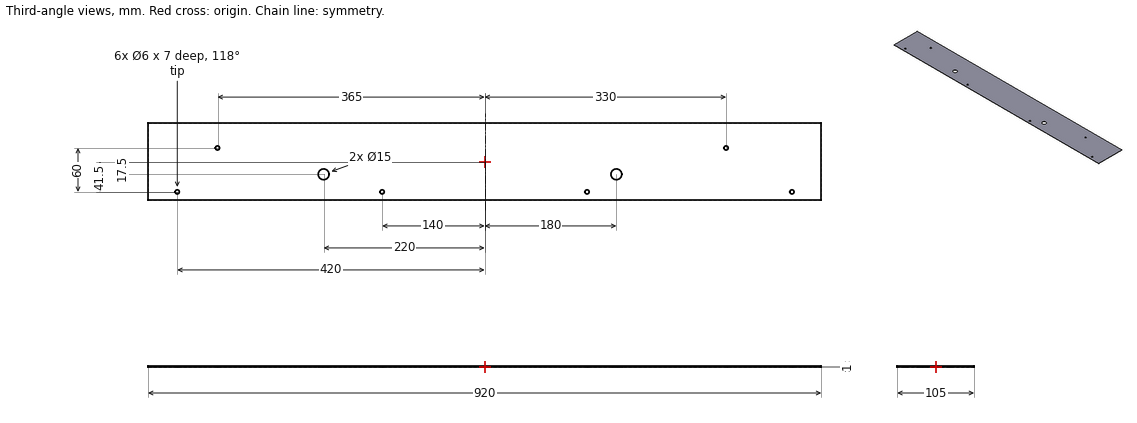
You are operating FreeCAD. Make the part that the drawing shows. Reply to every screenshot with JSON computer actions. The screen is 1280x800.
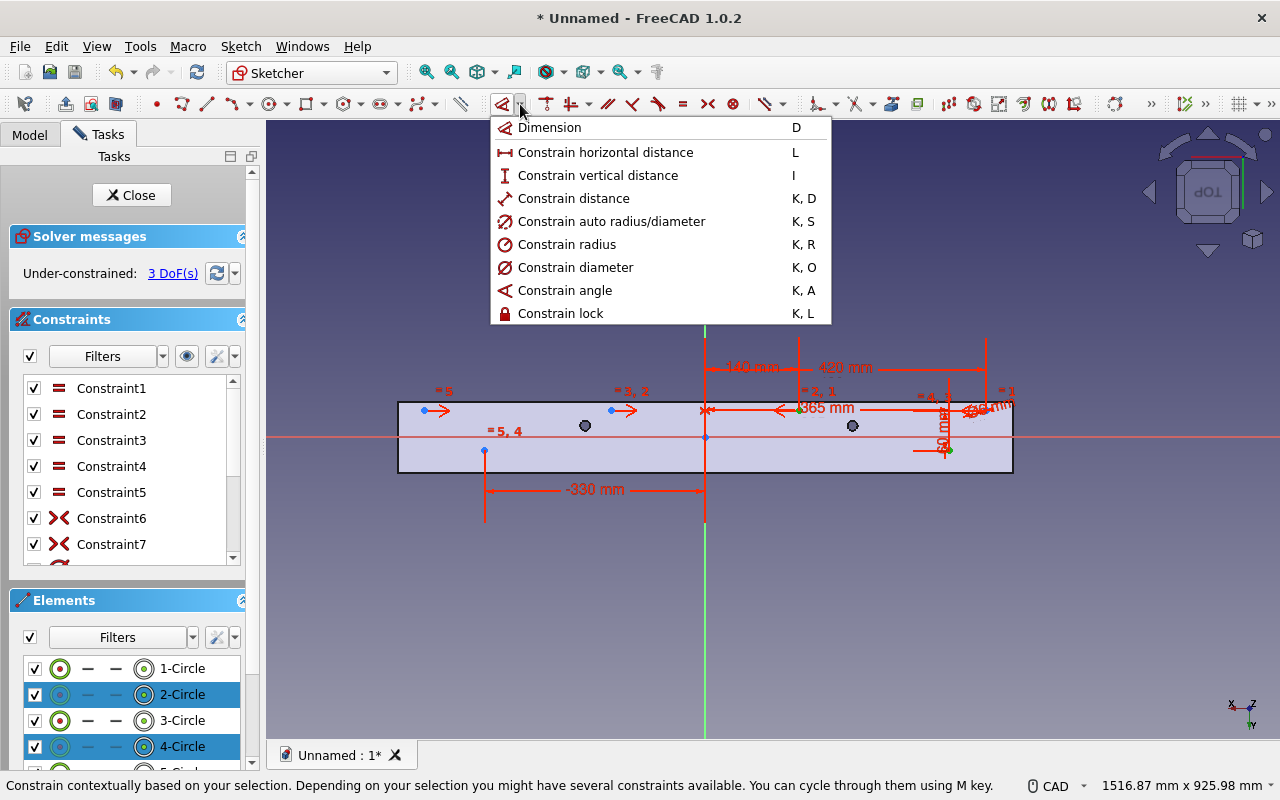
{"action": "left_click", "coordinate": [661, 176]}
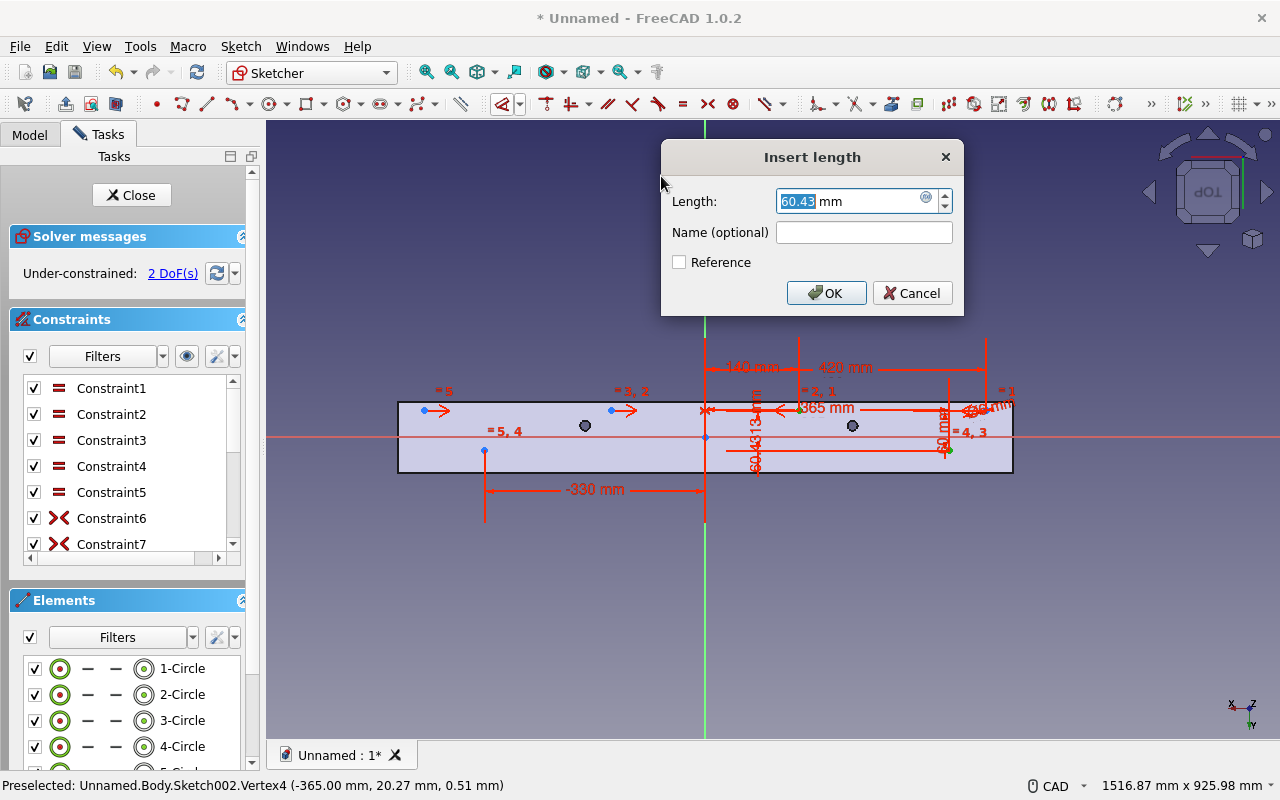
{"action": "type", "text": "60"}
{"action": "key", "text": "Return"}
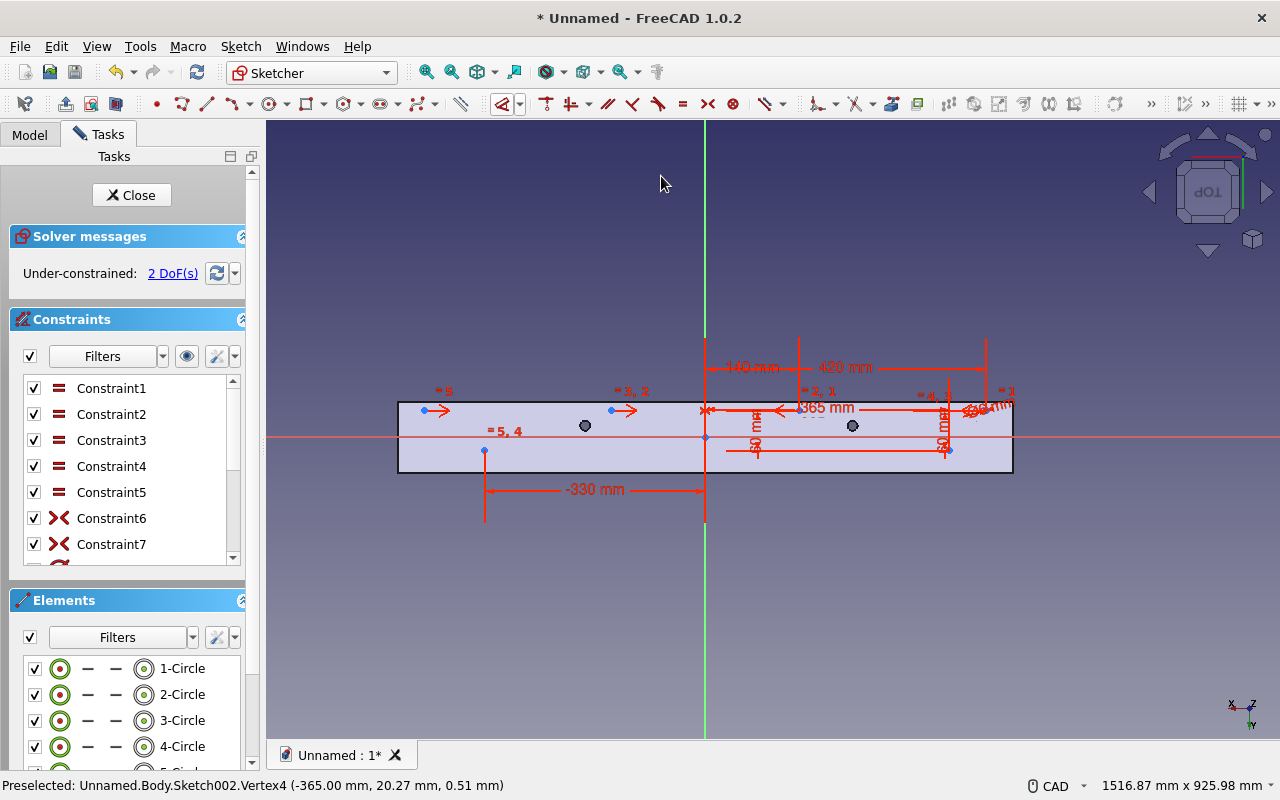
{"action": "left_click", "coordinate": [612, 411]}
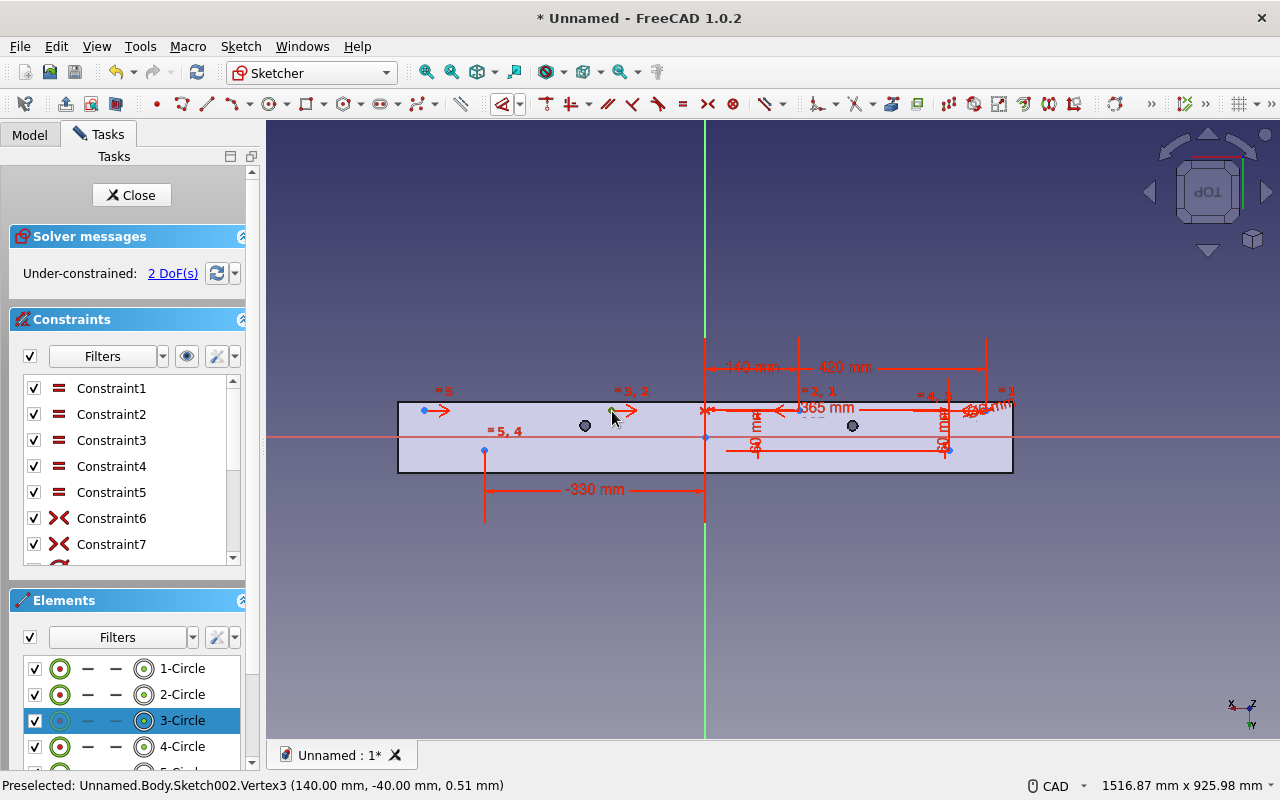
{"action": "left_click", "coordinate": [485, 450]}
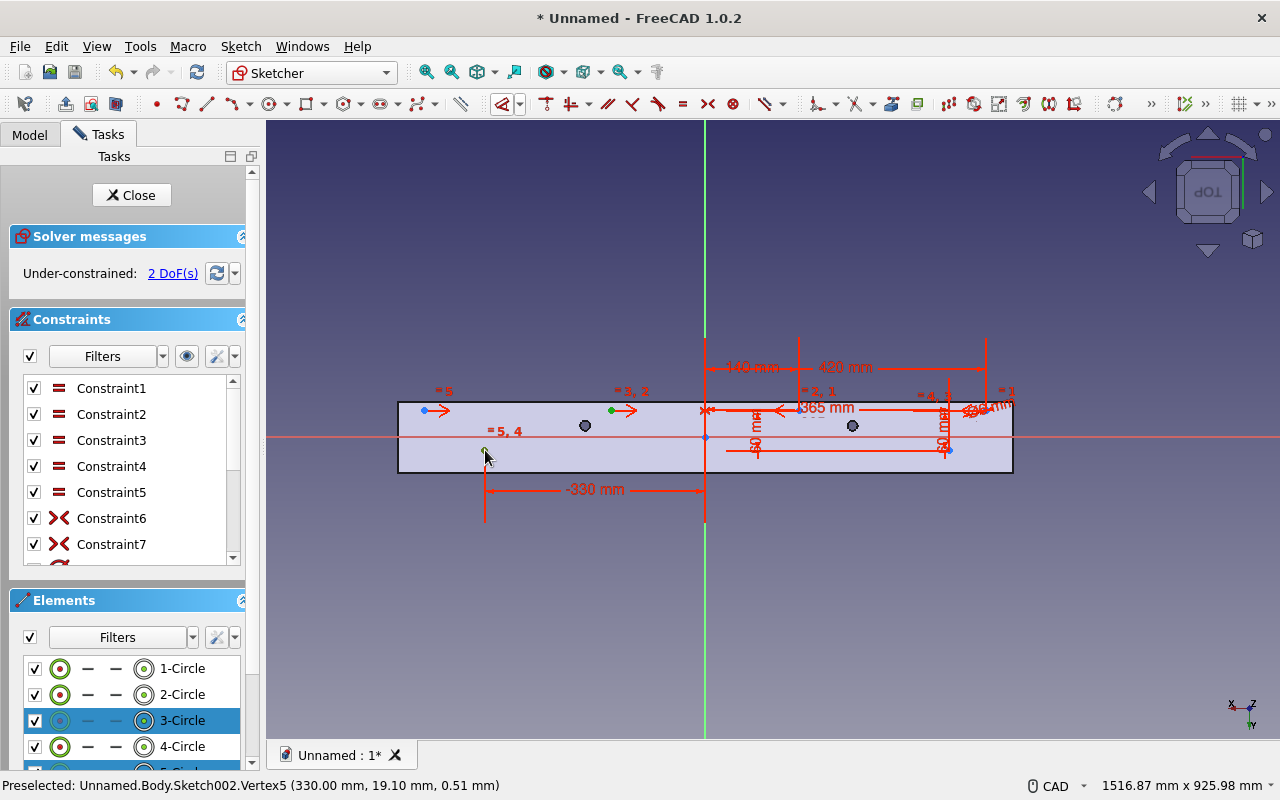
{"action": "left_click", "coordinate": [520, 104]}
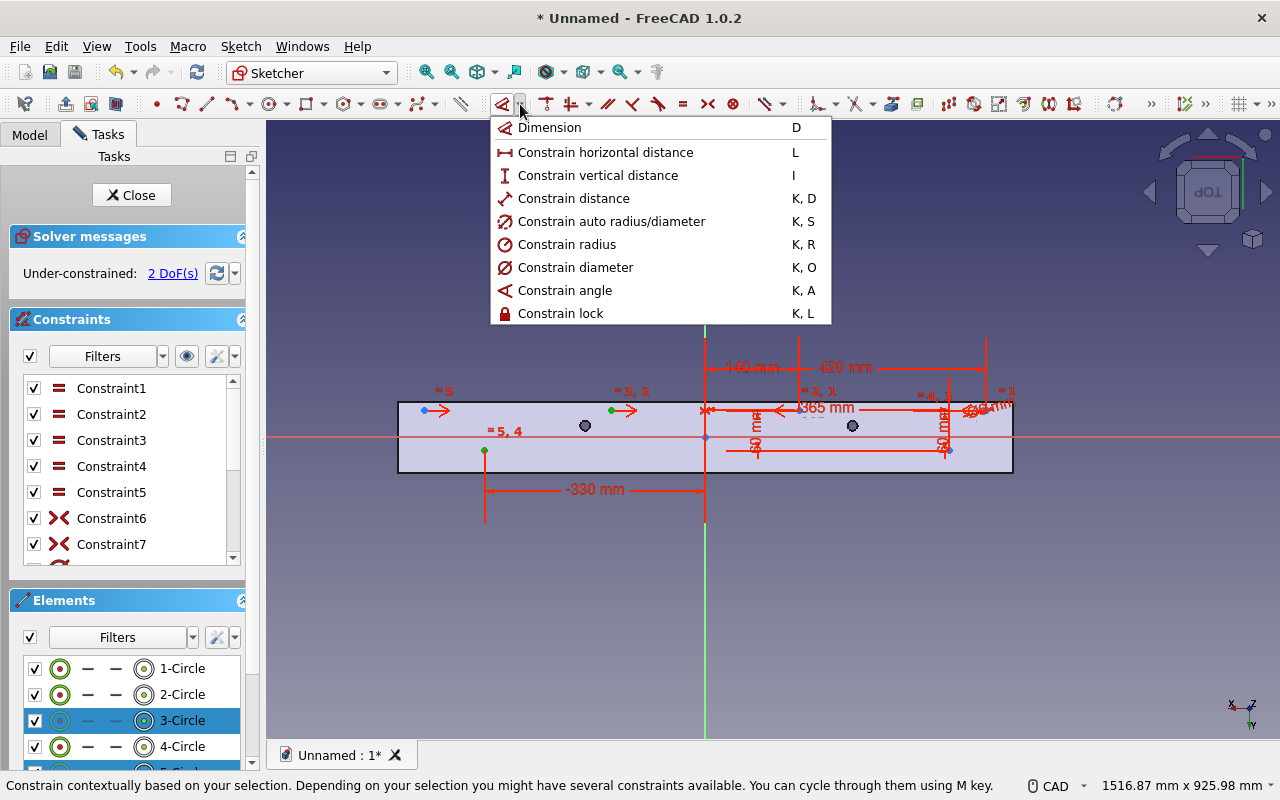
{"action": "left_click", "coordinate": [661, 176]}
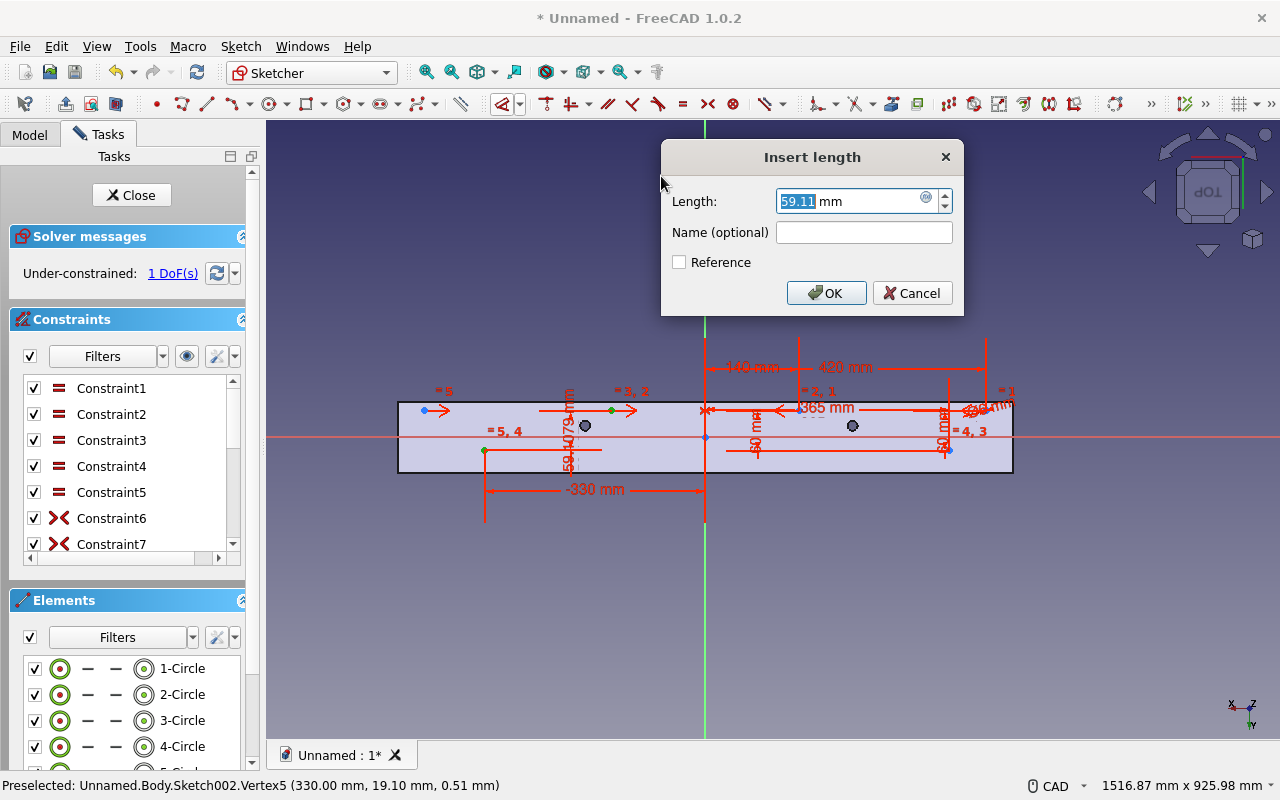
{"action": "type", "text": "60"}
{"action": "key", "text": "Return"}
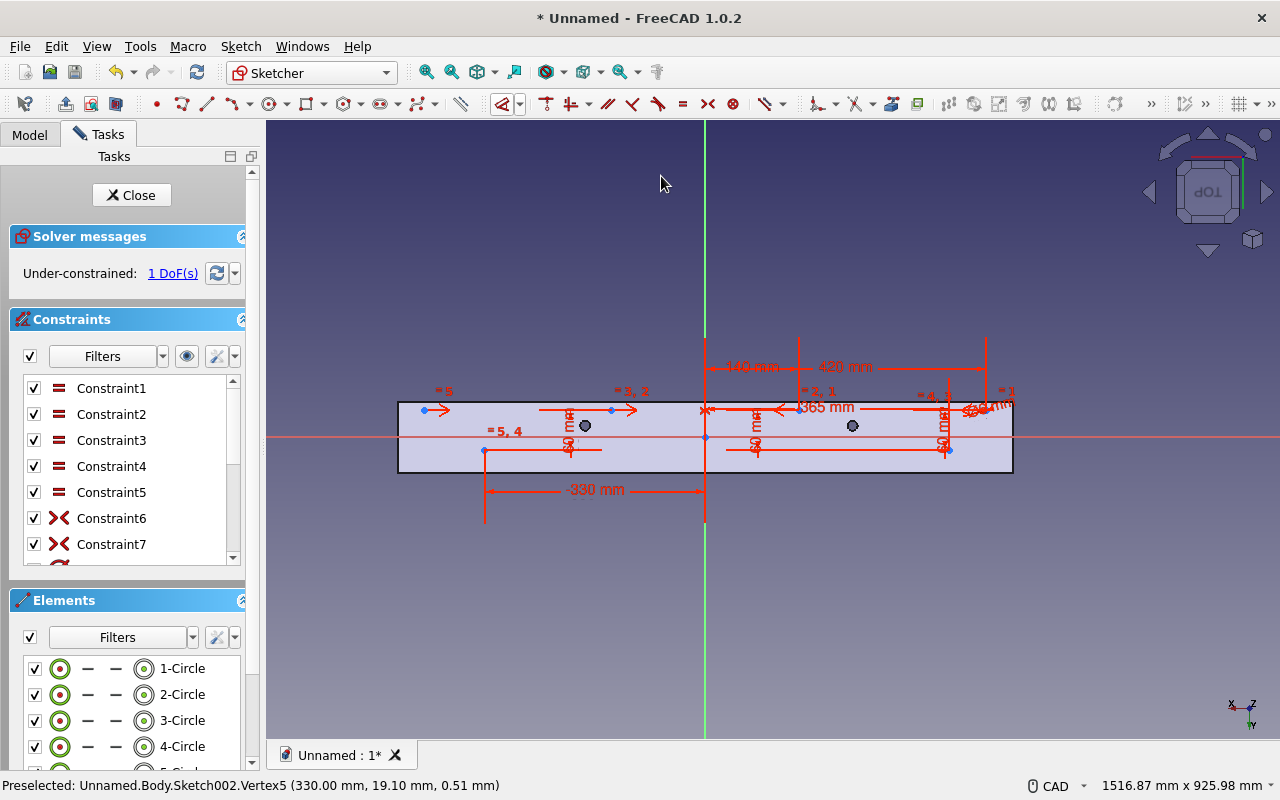
{"action": "scroll", "coordinate": [986, 410], "scroll_direction": "up", "scroll_amount": 2}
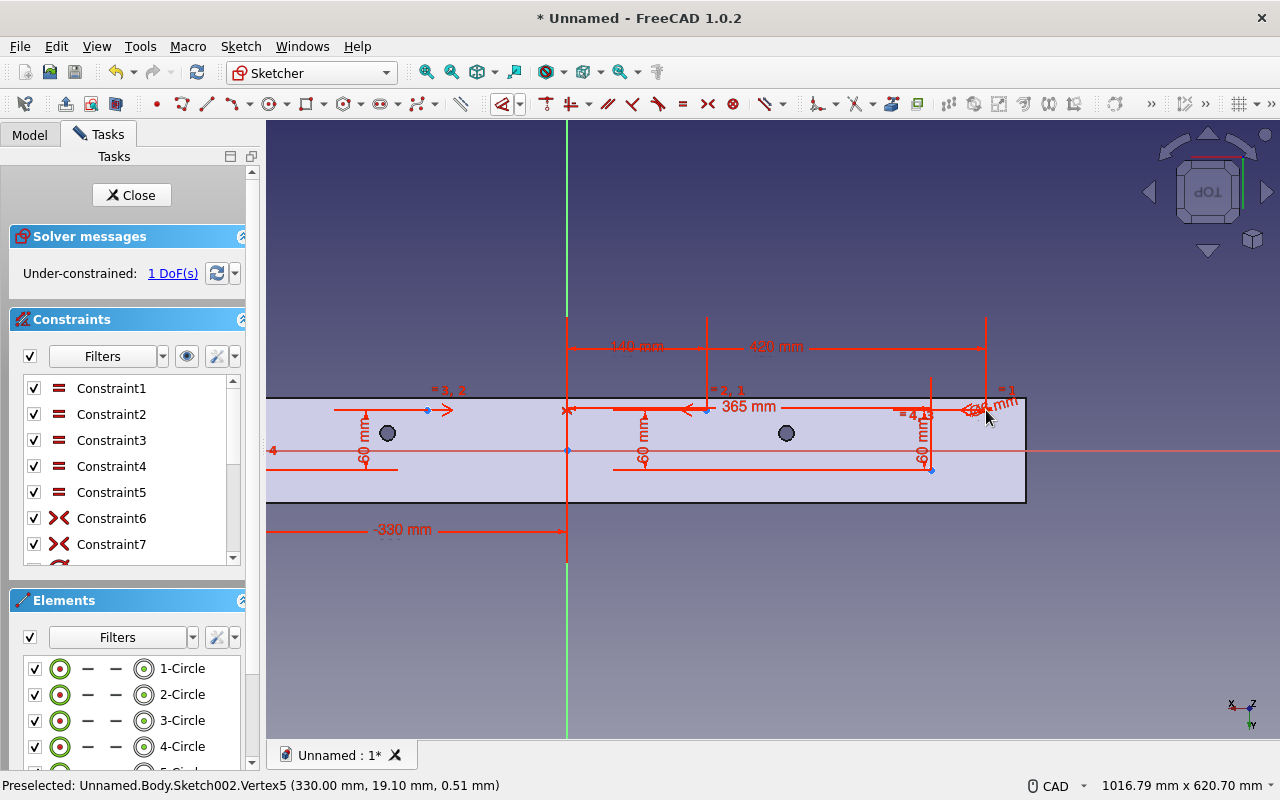
{"action": "left_click", "coordinate": [986, 410]}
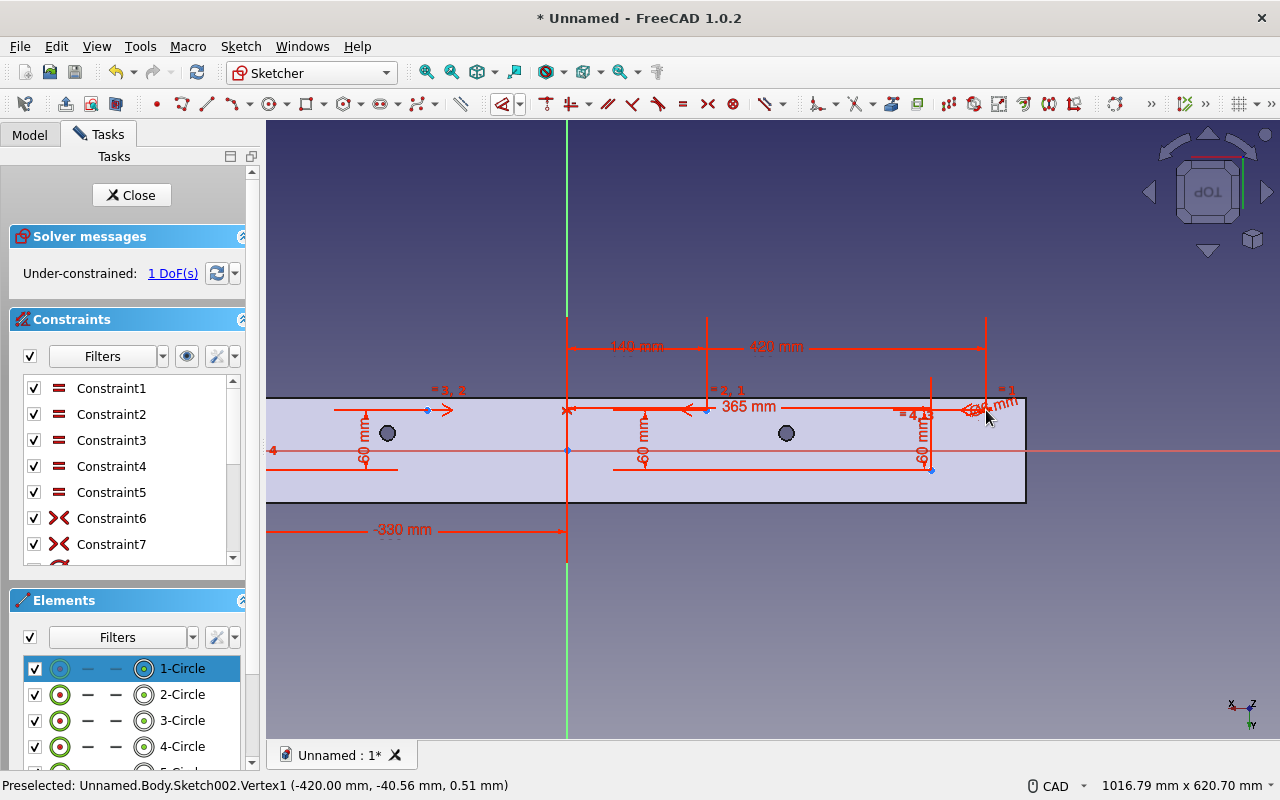
{"action": "key", "text": "i"}